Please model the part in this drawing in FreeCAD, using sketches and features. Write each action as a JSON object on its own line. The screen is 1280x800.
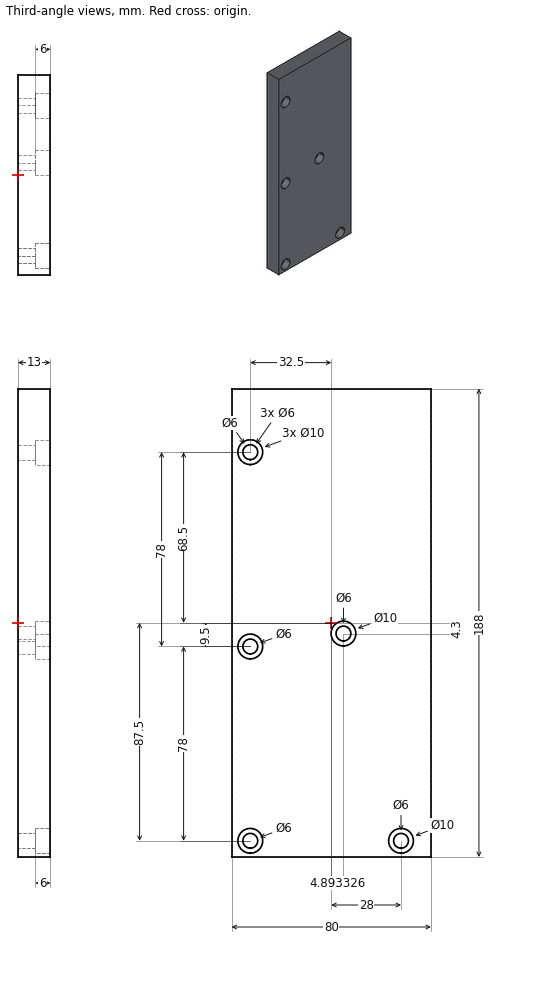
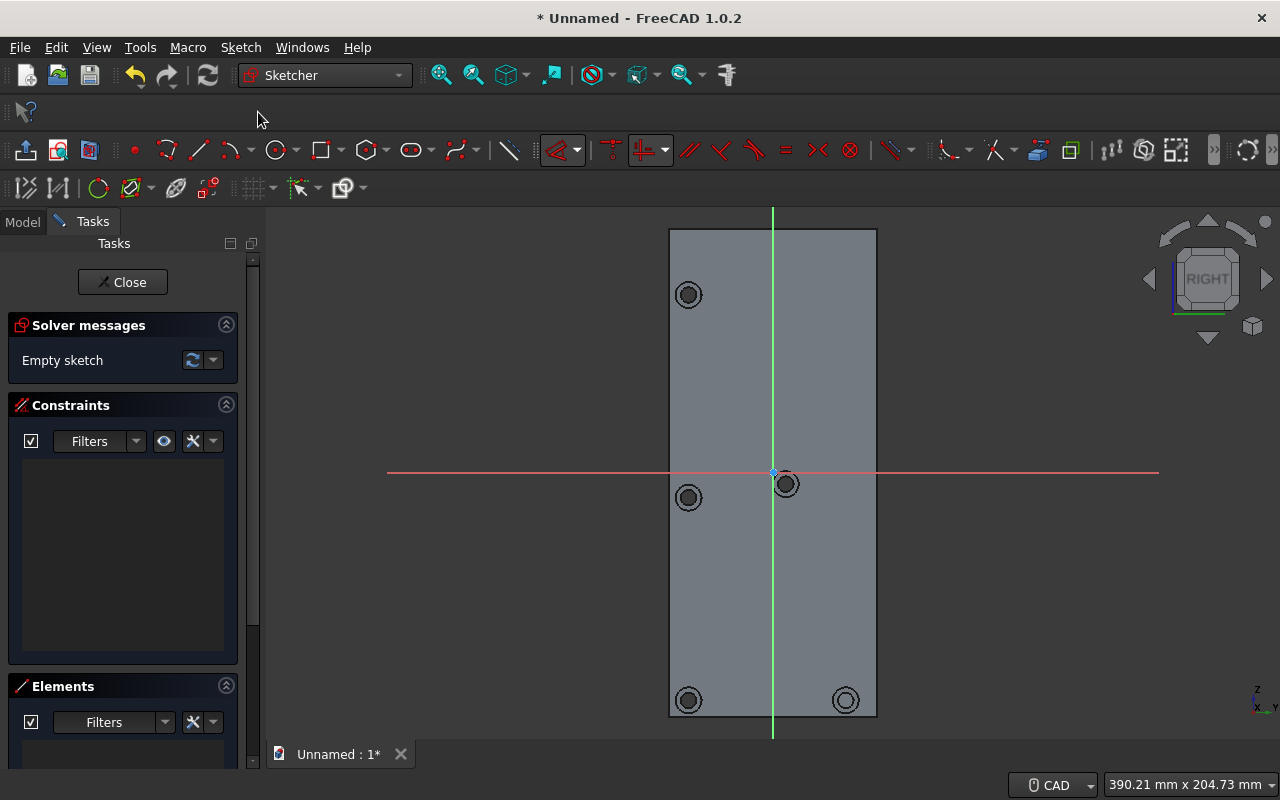
{"action": "scroll", "coordinate": [853, 711], "scroll_direction": "up", "scroll_amount": 15}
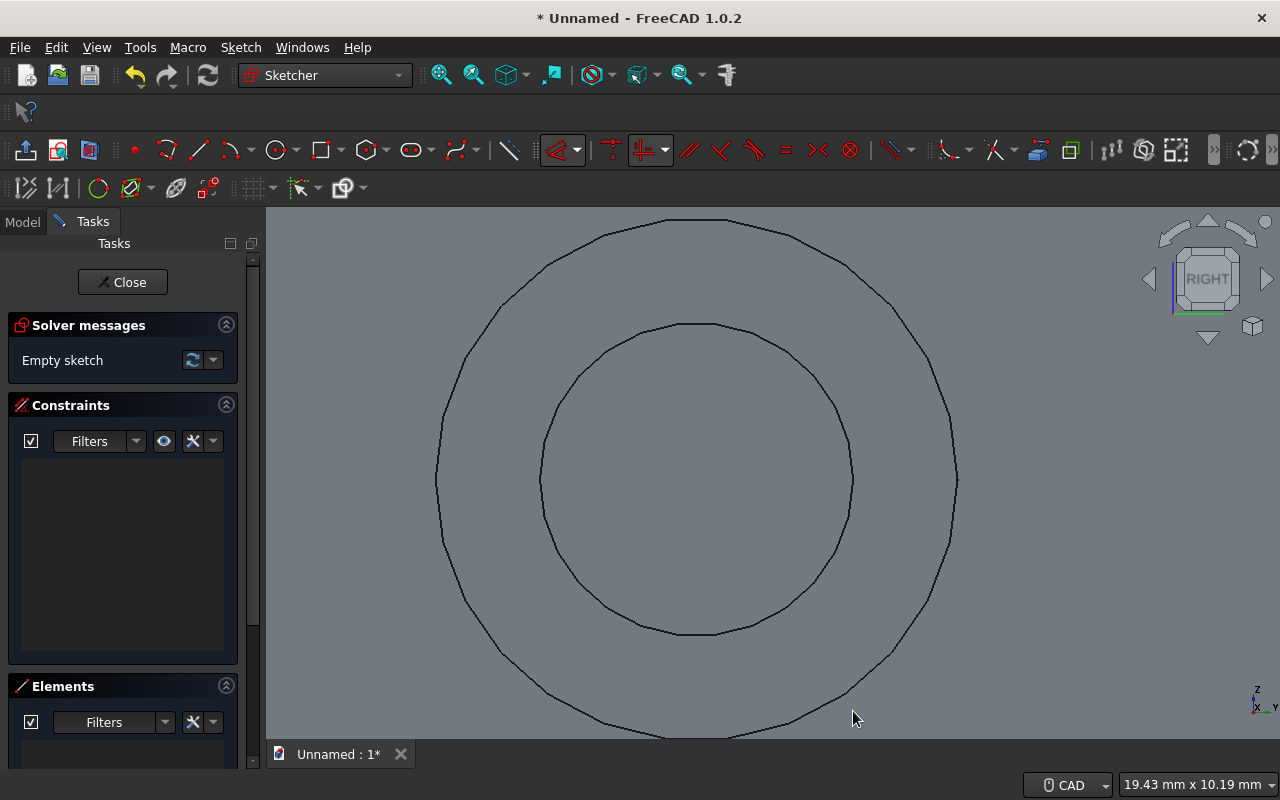
{"action": "left_click", "coordinate": [276, 150]}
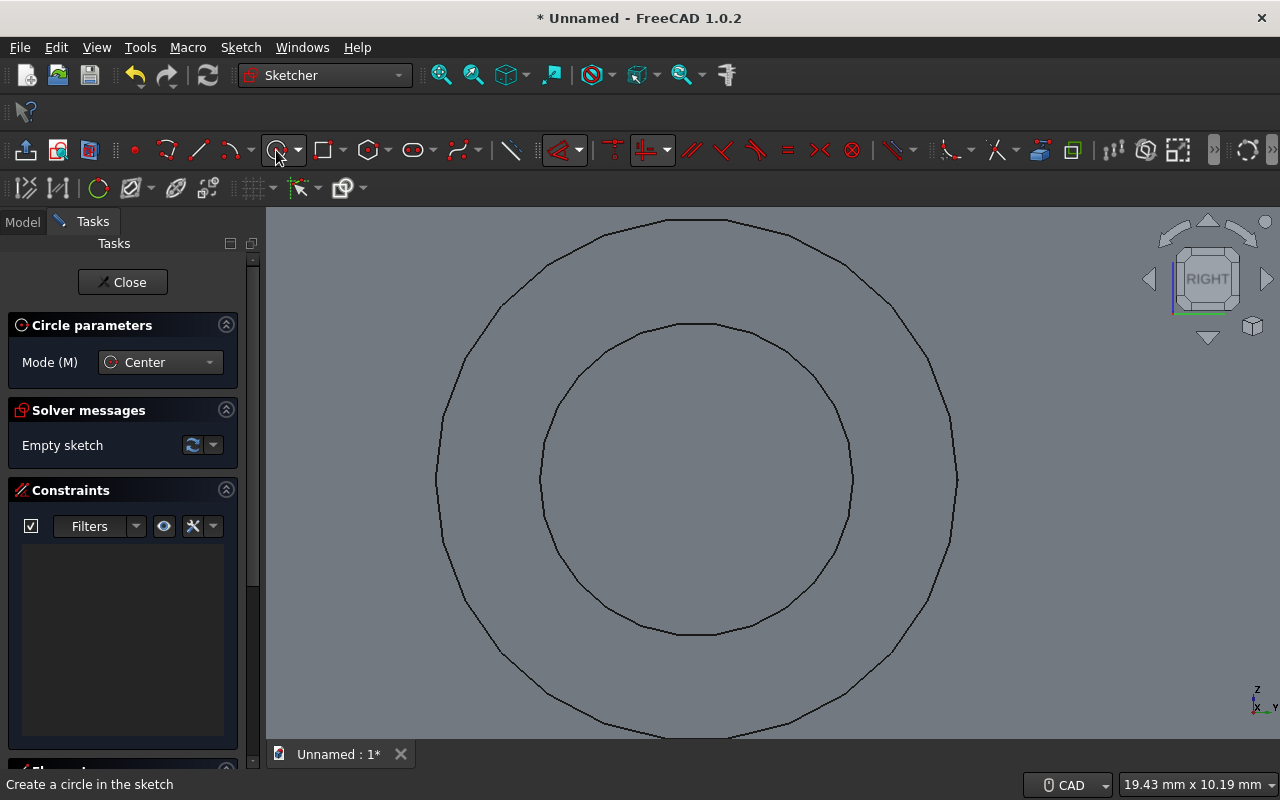
{"action": "left_click", "coordinate": [697, 480]}
{"action": "left_click", "coordinate": [807, 369]}
{"action": "key", "text": "Escape"}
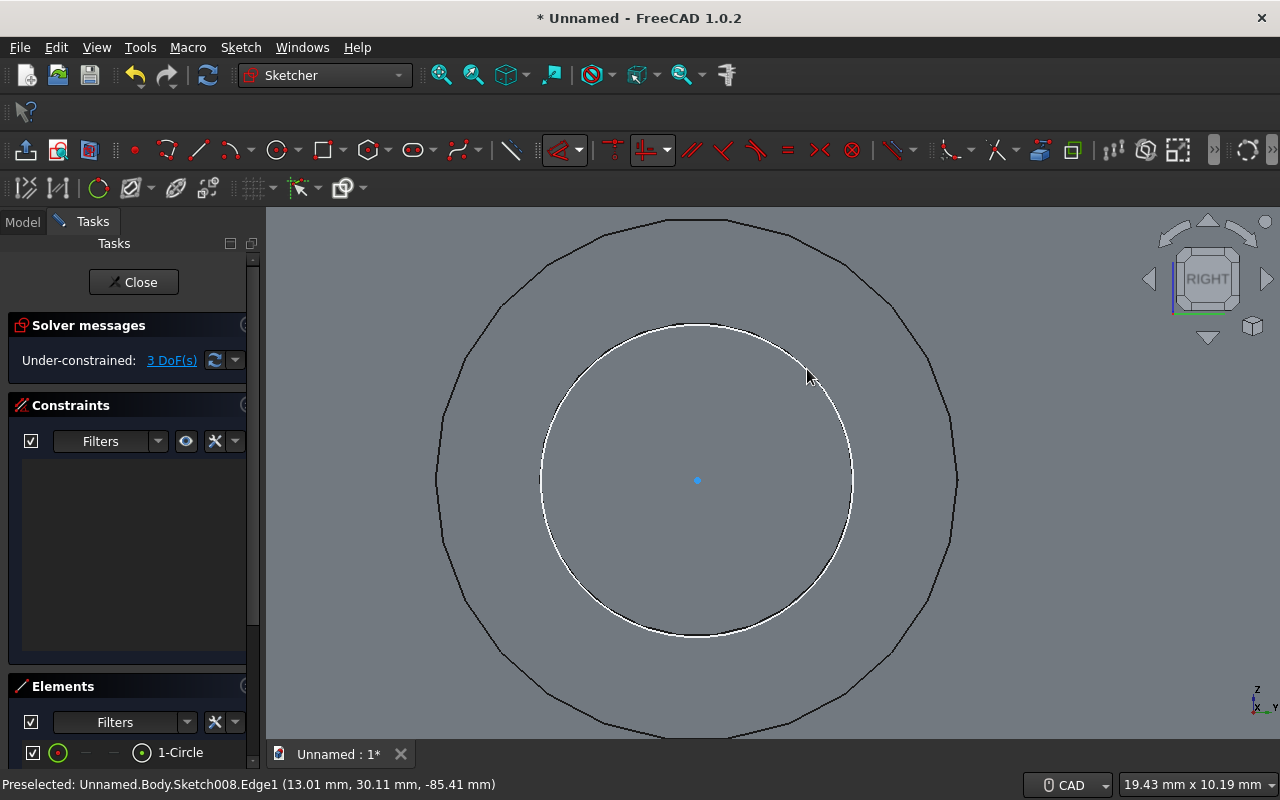
{"action": "left_click", "coordinate": [807, 370]}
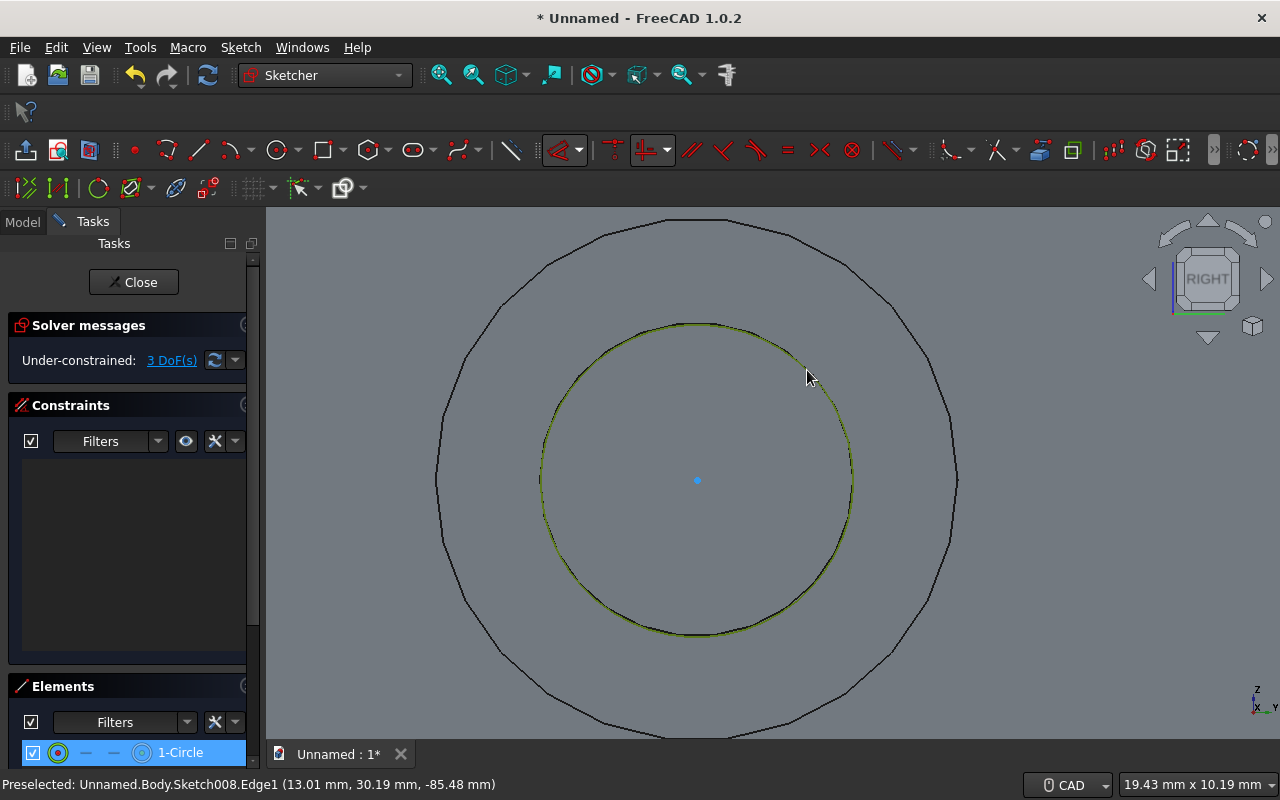
{"action": "left_click", "coordinate": [582, 150]}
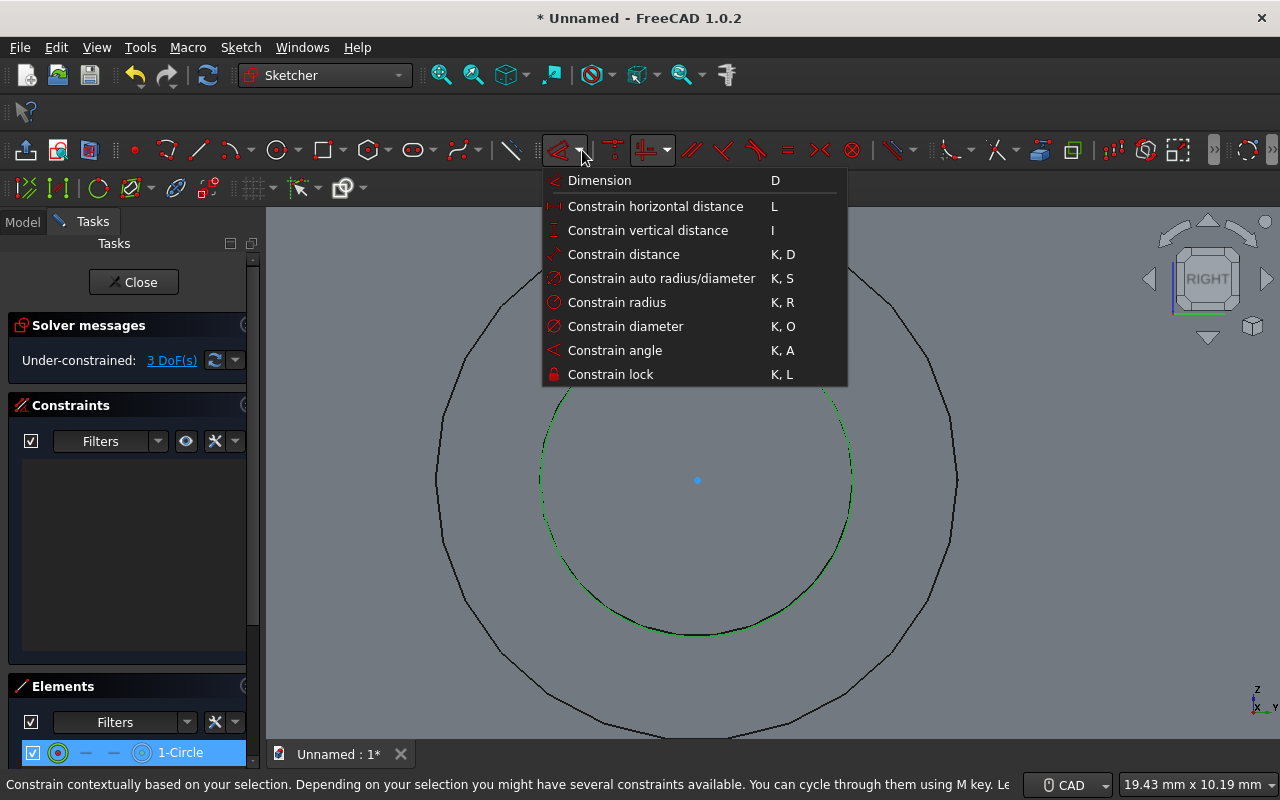
{"action": "left_click", "coordinate": [695, 326]}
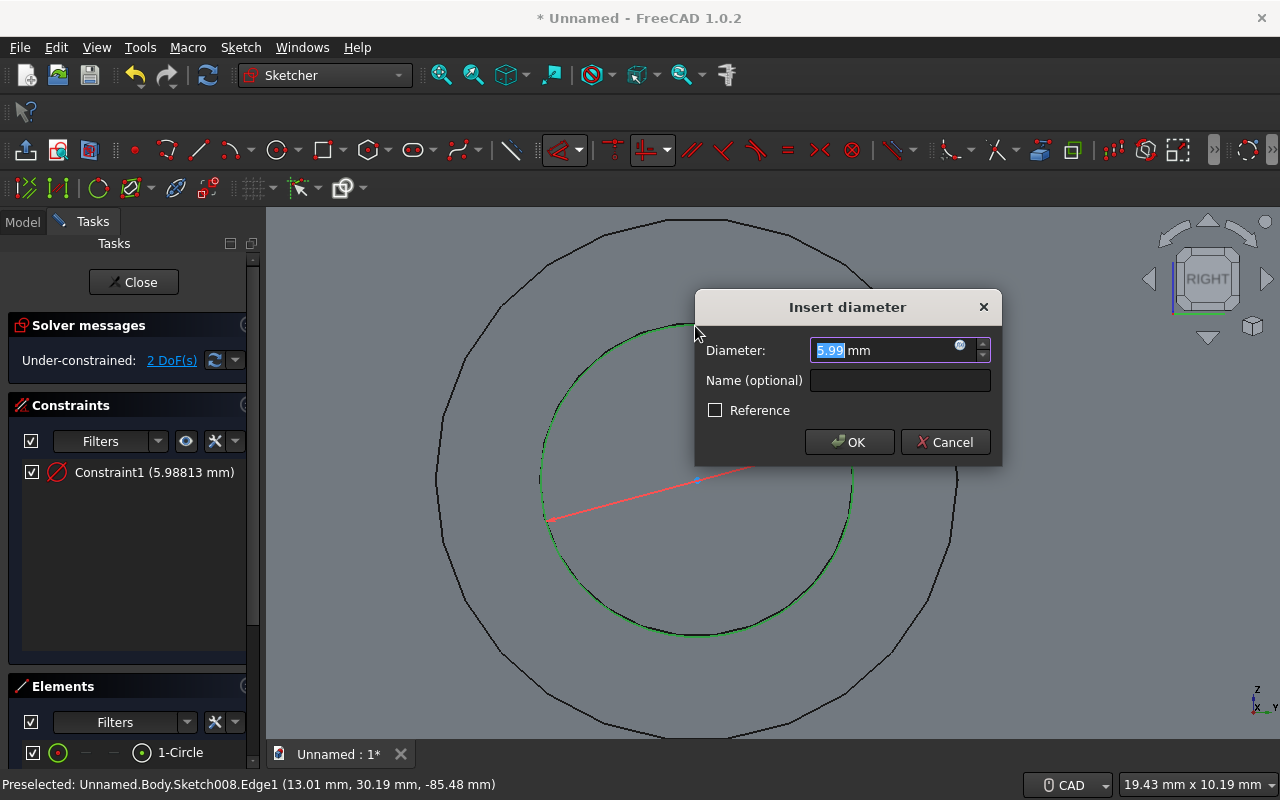
{"action": "type", "text": "6"}
{"action": "key", "text": "Return"}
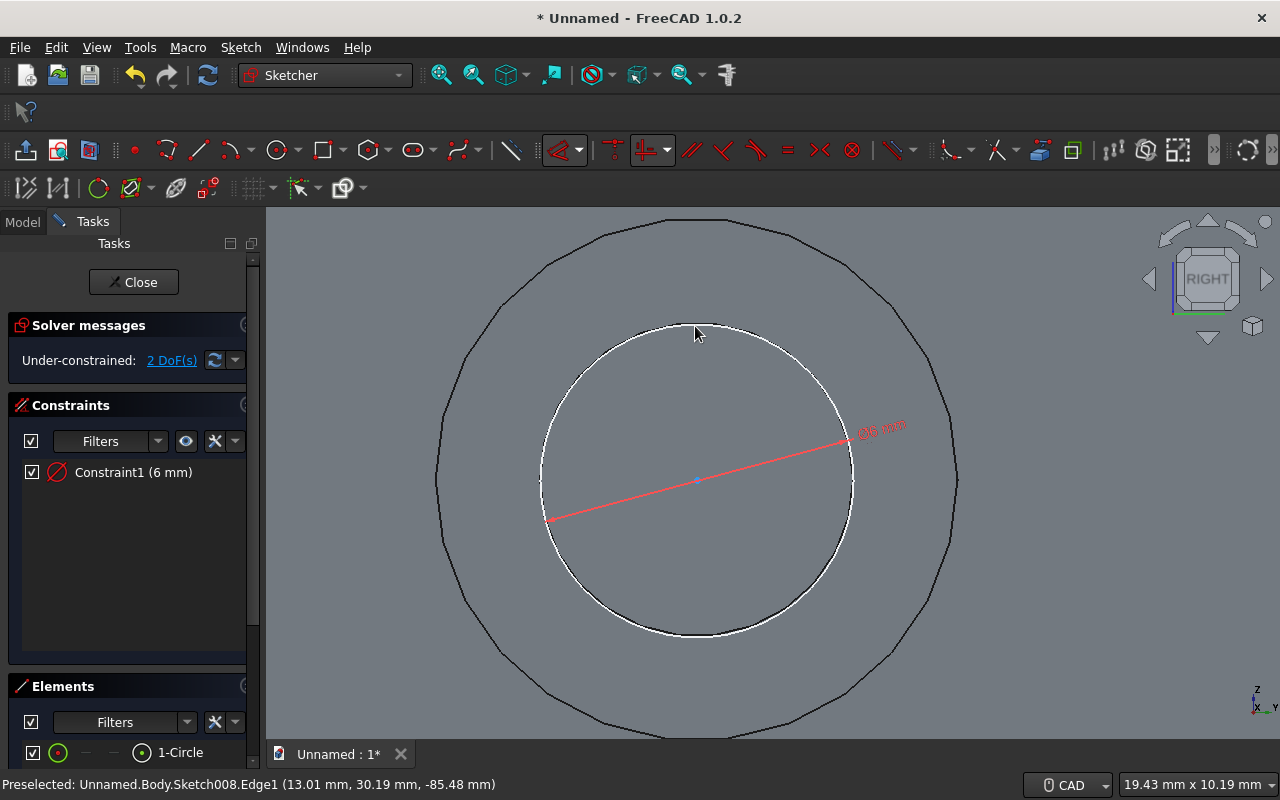
{"action": "left_click", "coordinate": [697, 481]}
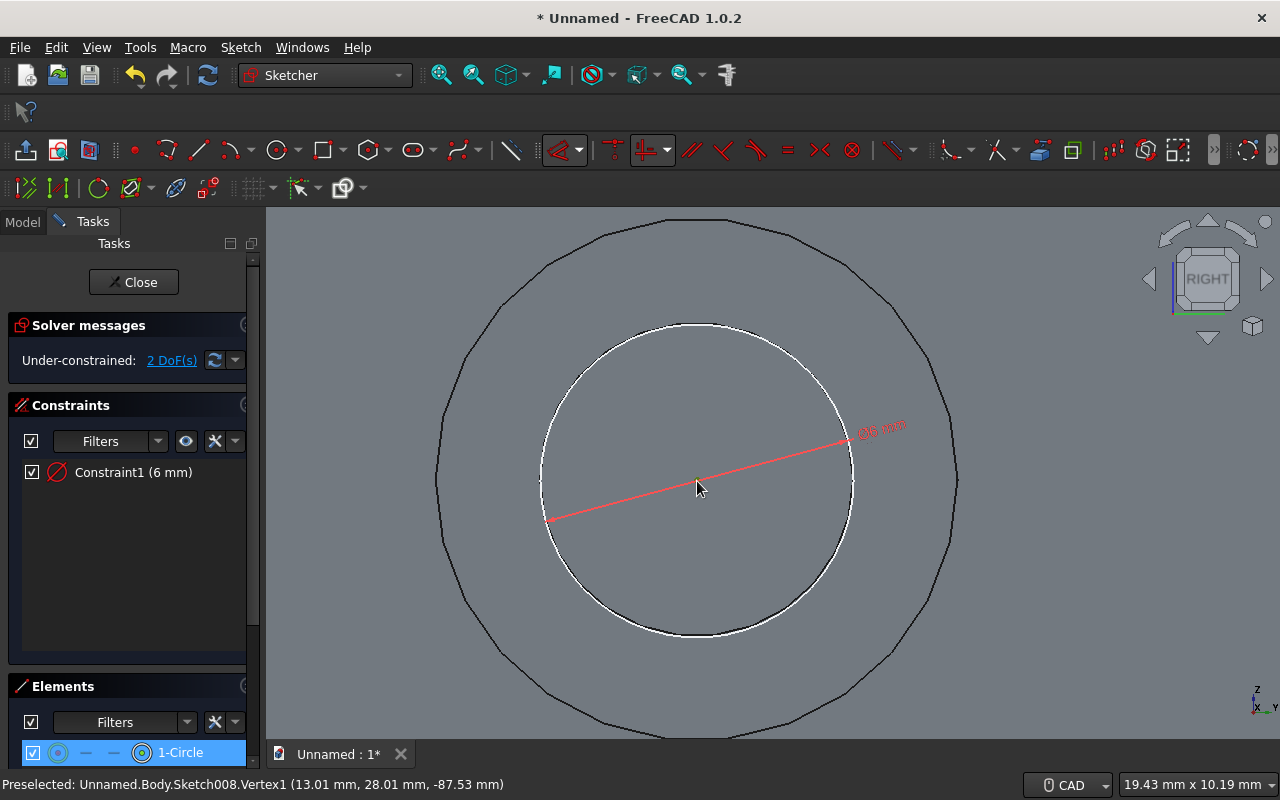
{"action": "left_click", "coordinate": [582, 150]}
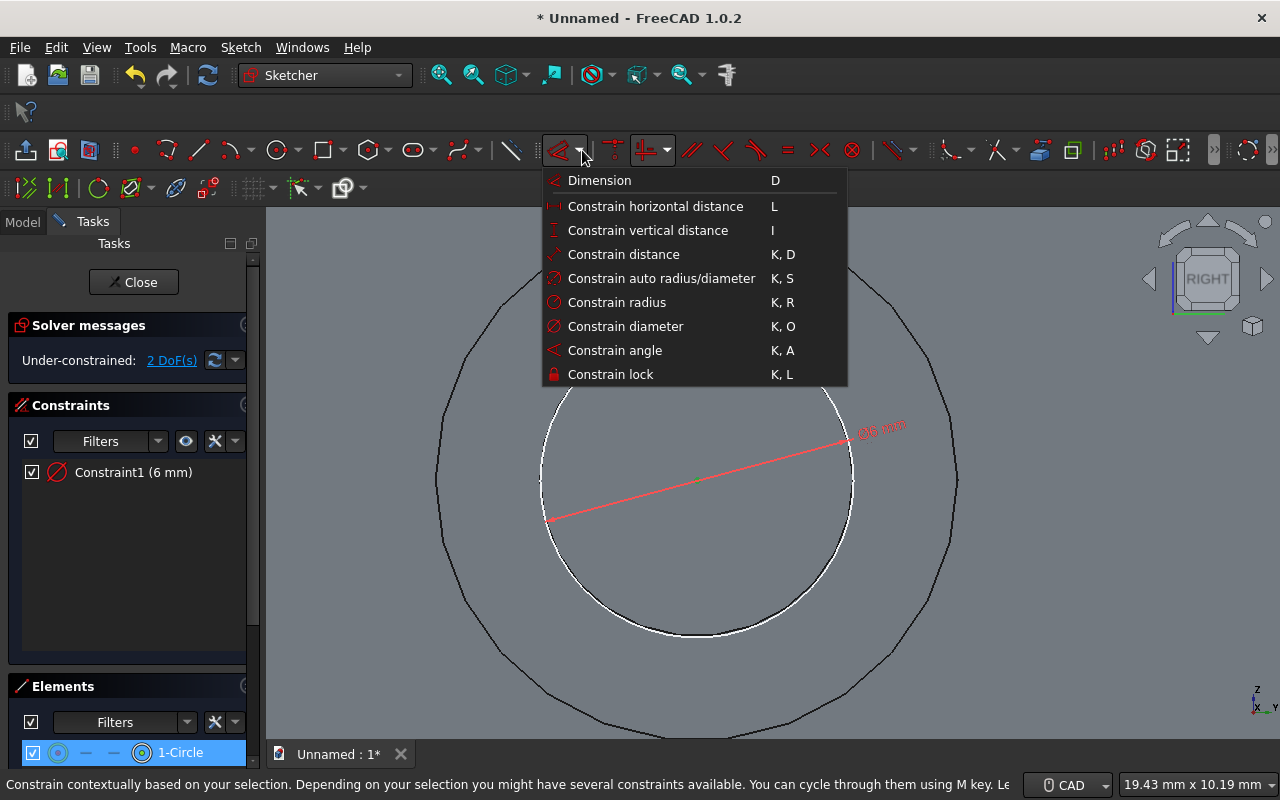
{"action": "left_click", "coordinate": [695, 206]}